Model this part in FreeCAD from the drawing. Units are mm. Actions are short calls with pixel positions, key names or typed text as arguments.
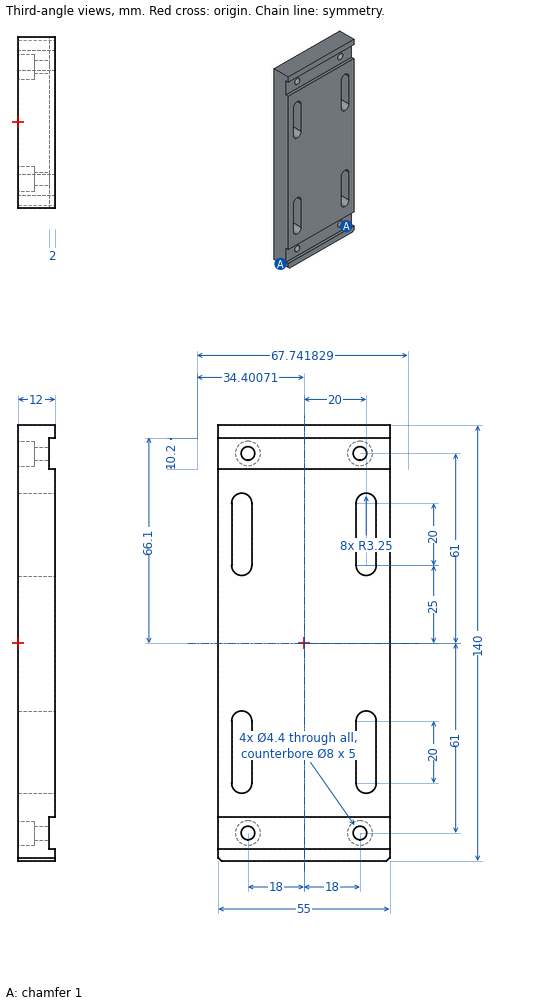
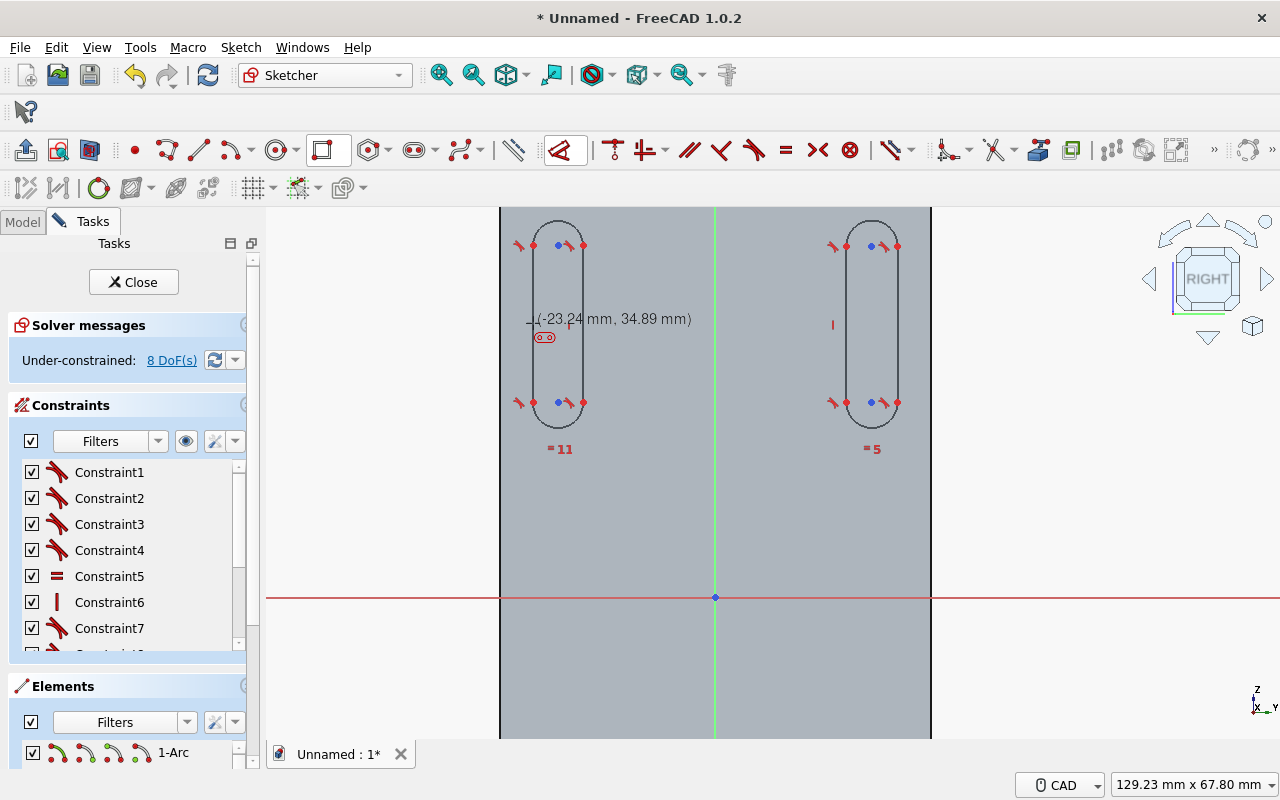
scroll(696, 371, down, 4)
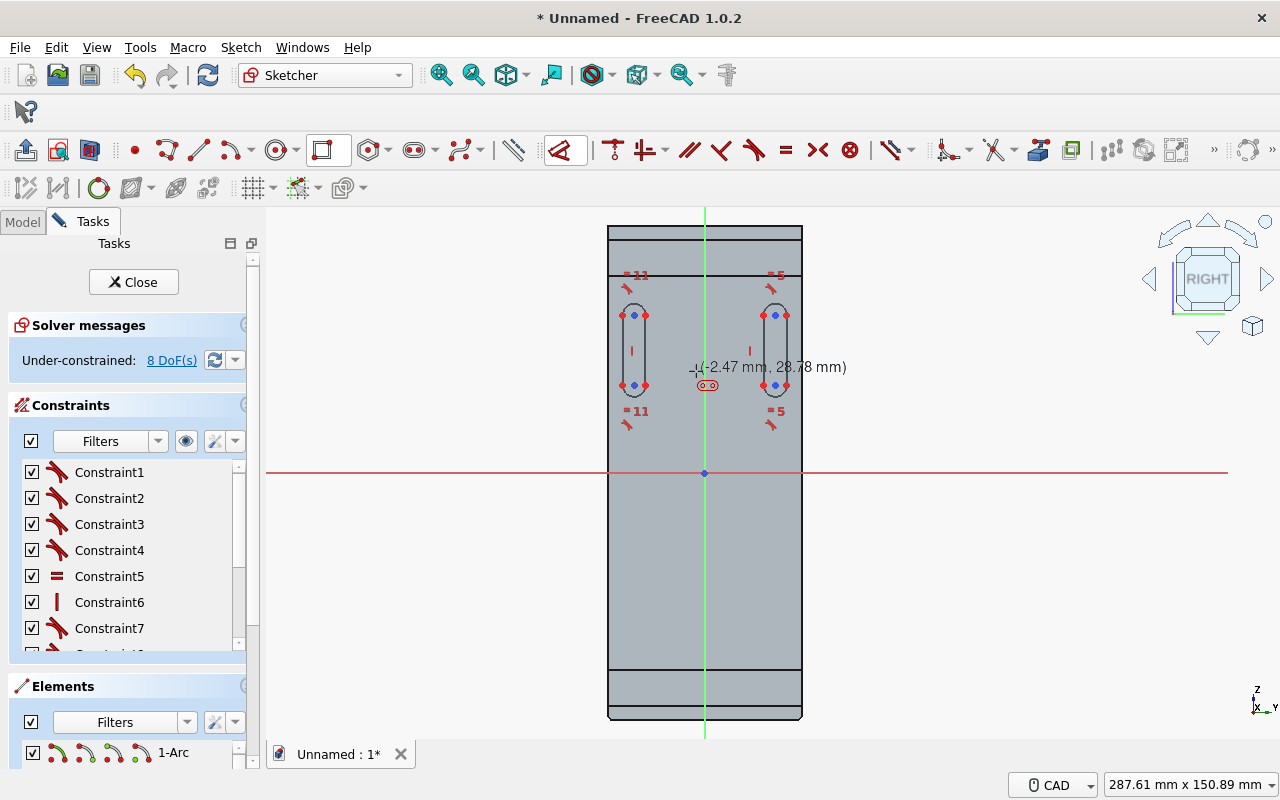
scroll(775, 632, up, 4)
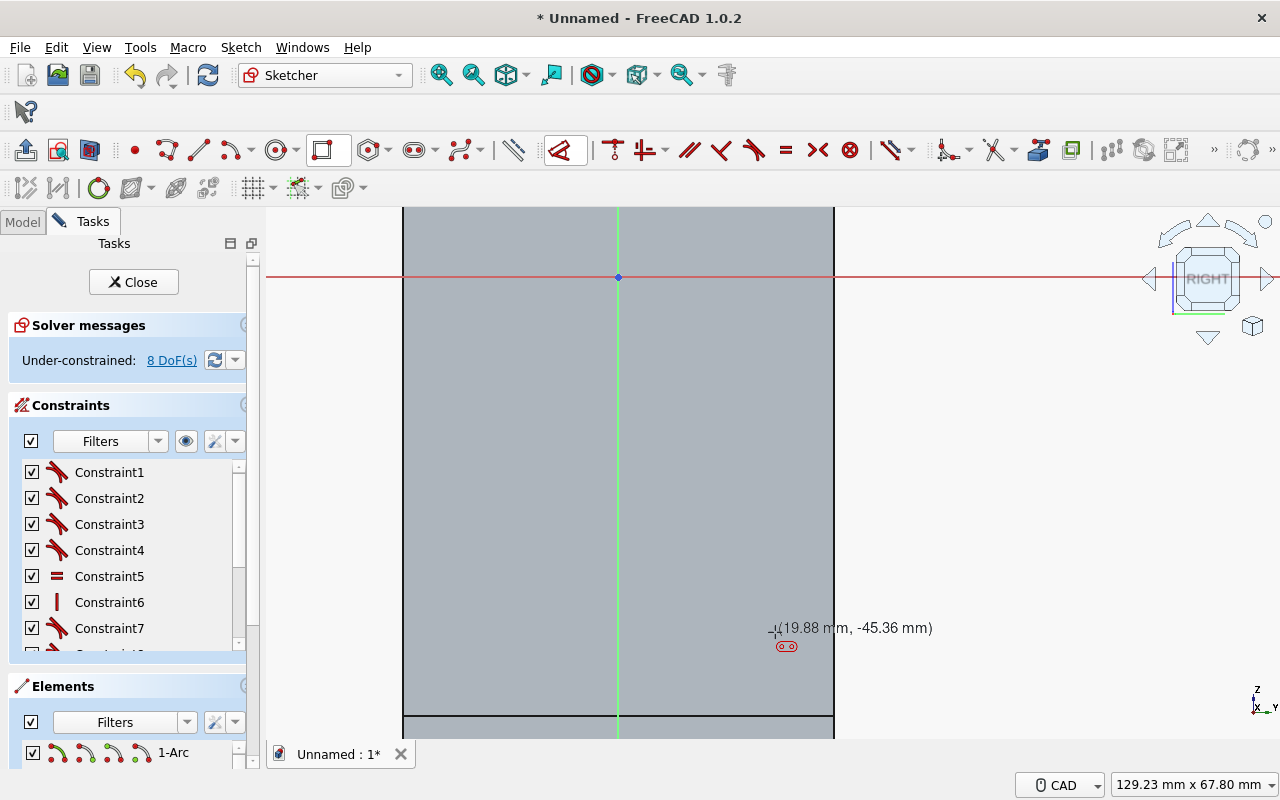
click(775, 630)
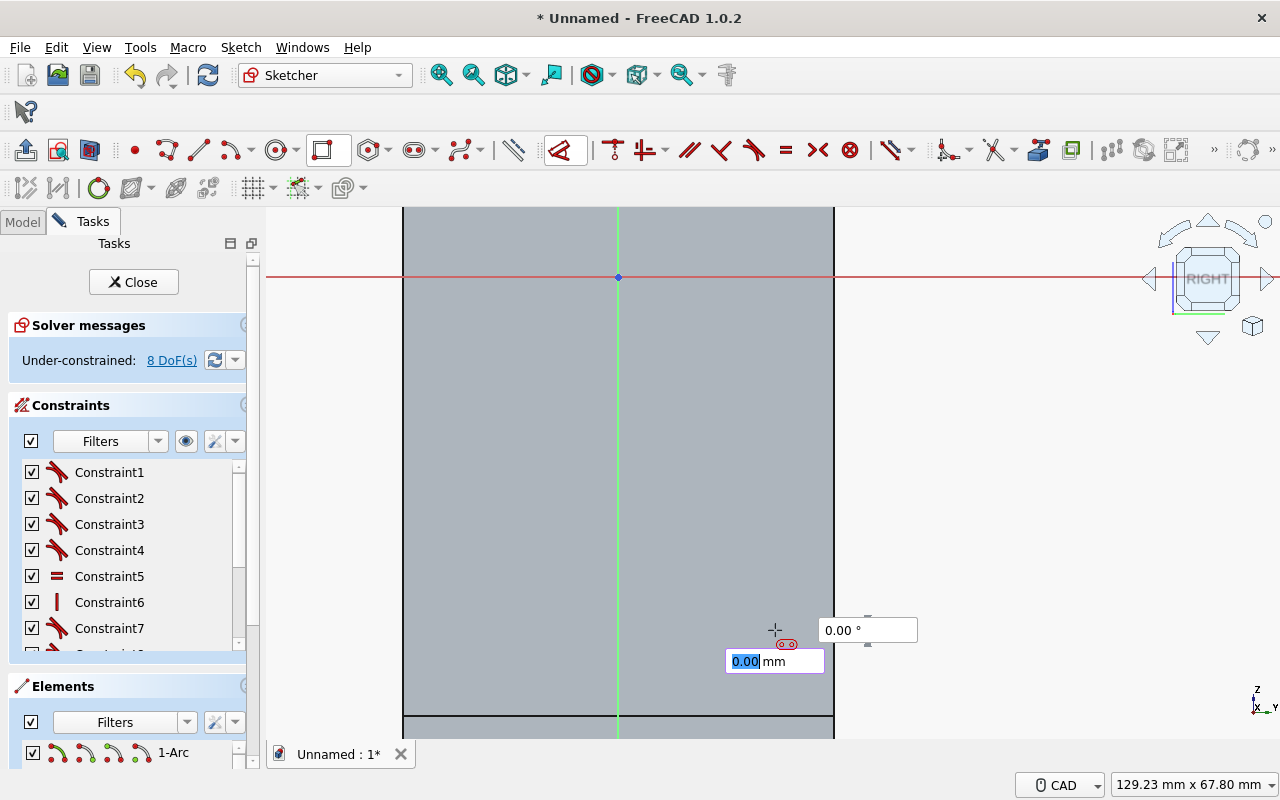
click(775, 473)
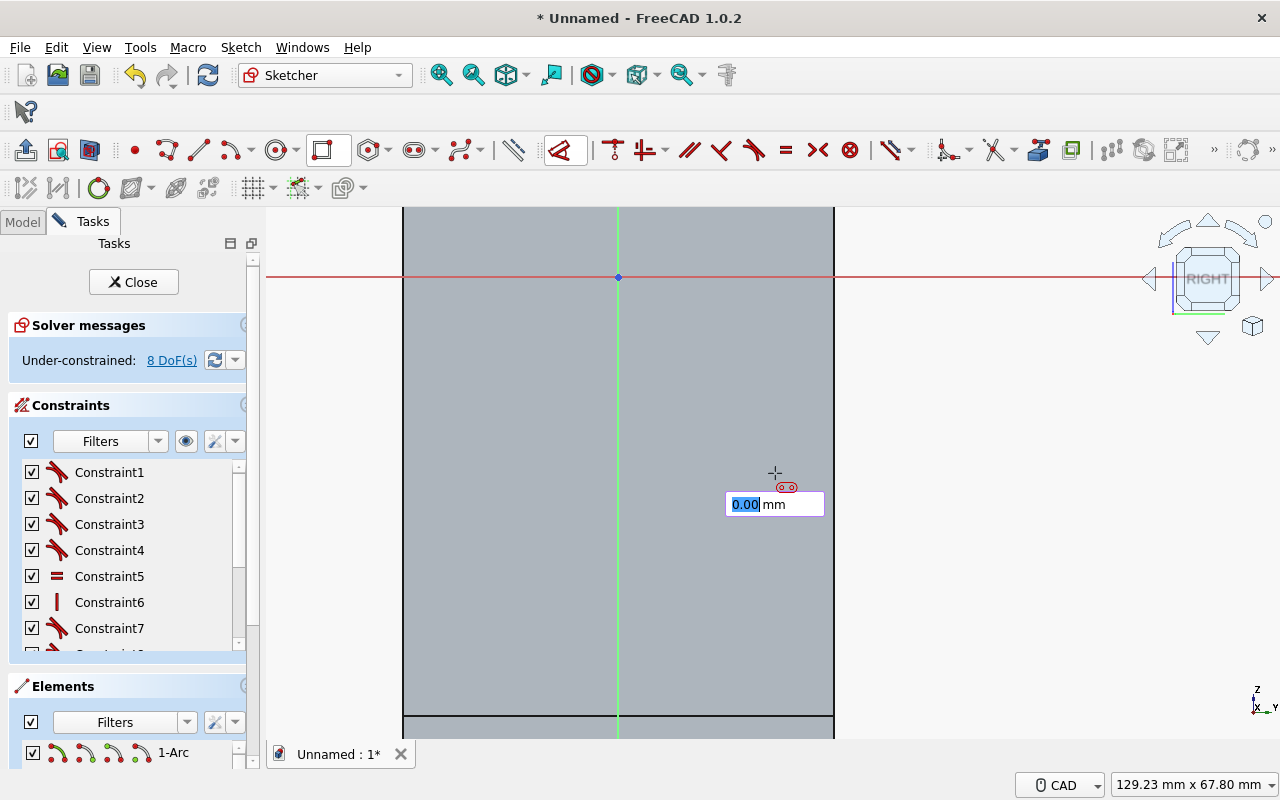
click(801, 552)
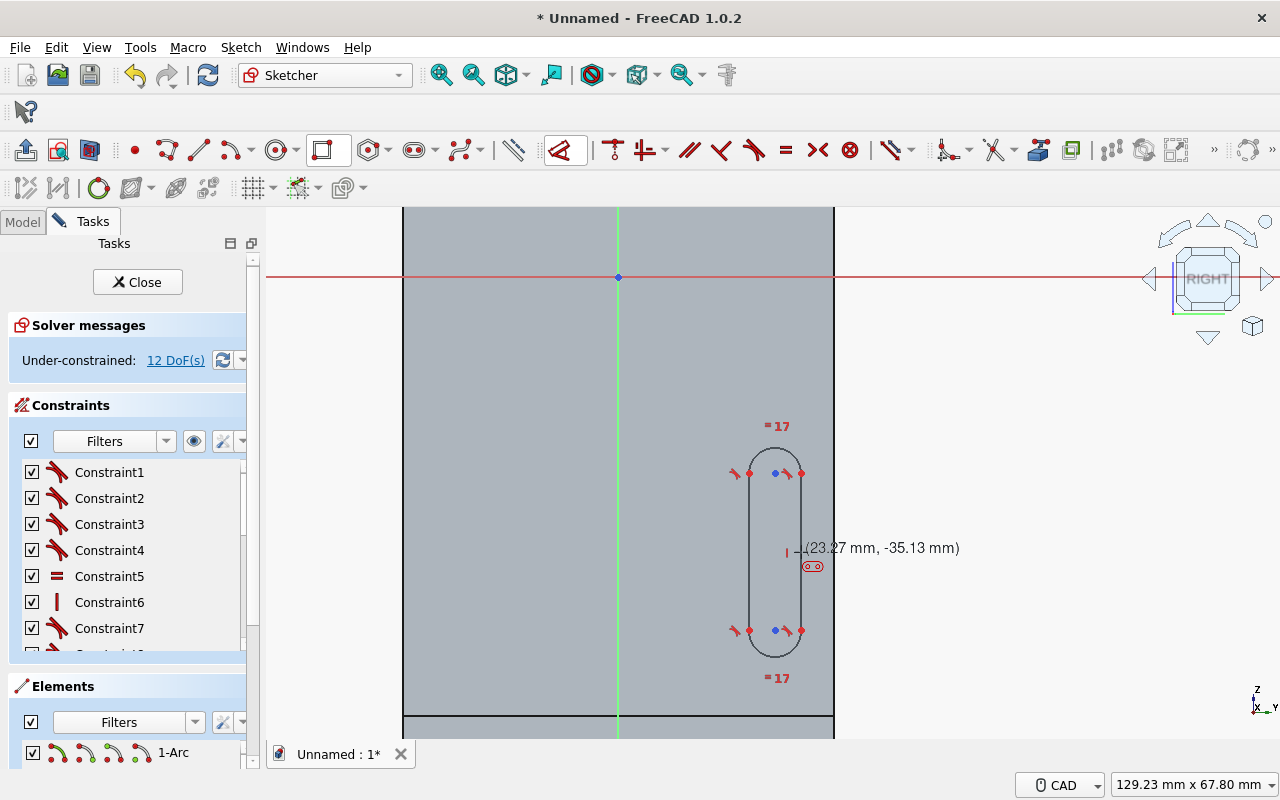
click(461, 630)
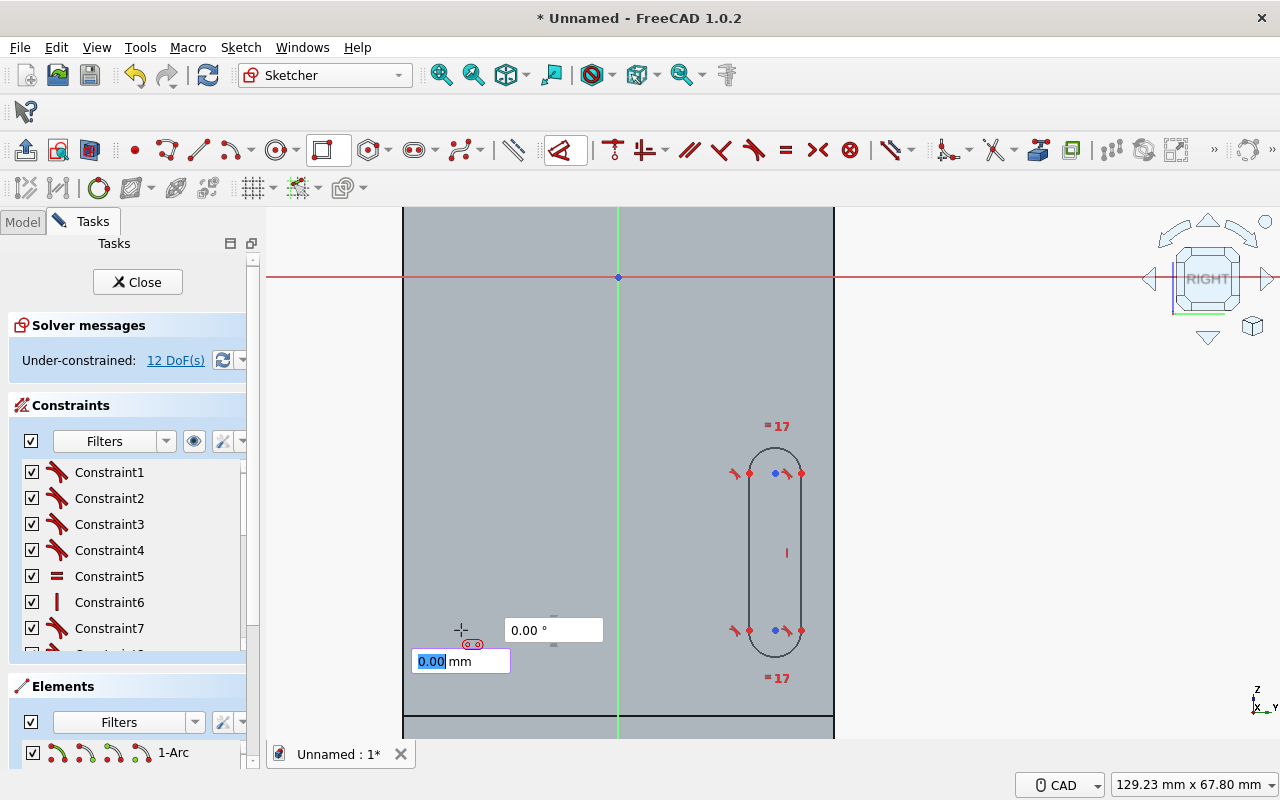
click(461, 473)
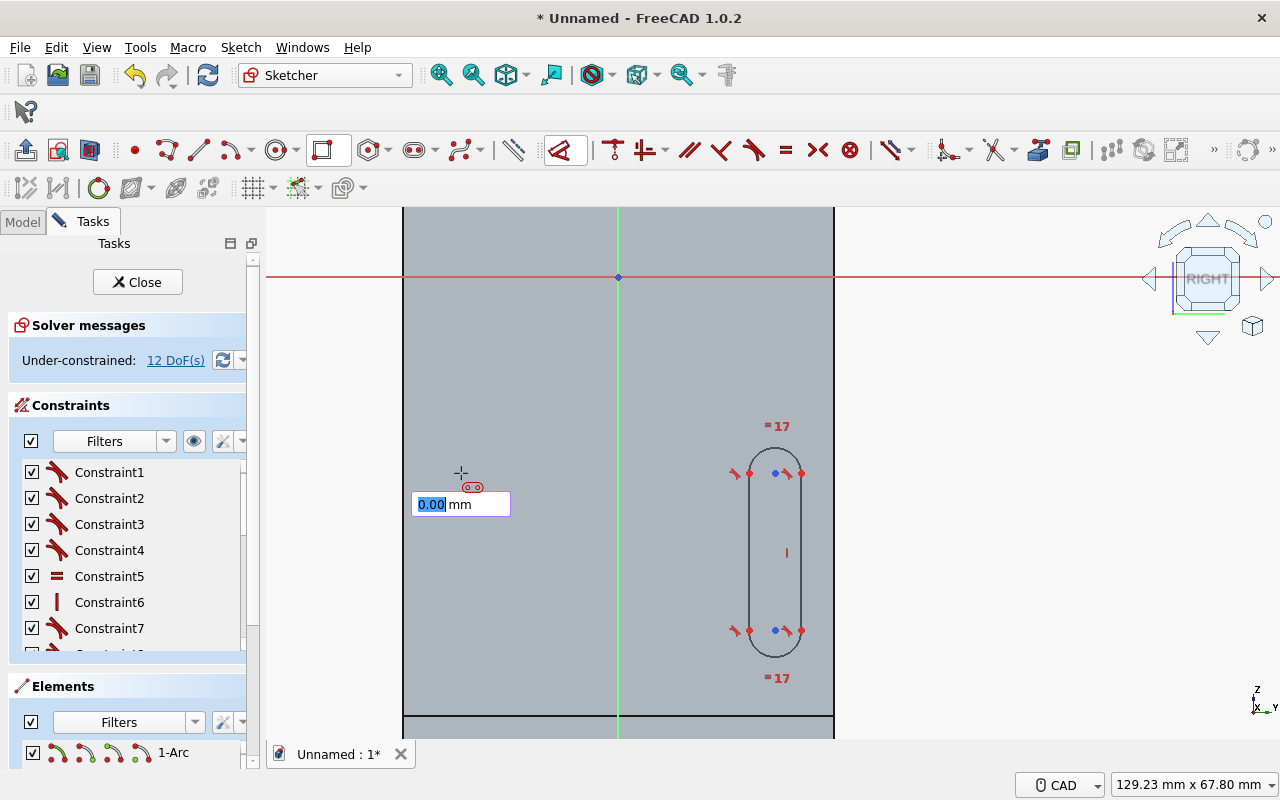
click(436, 552)
key(Escape)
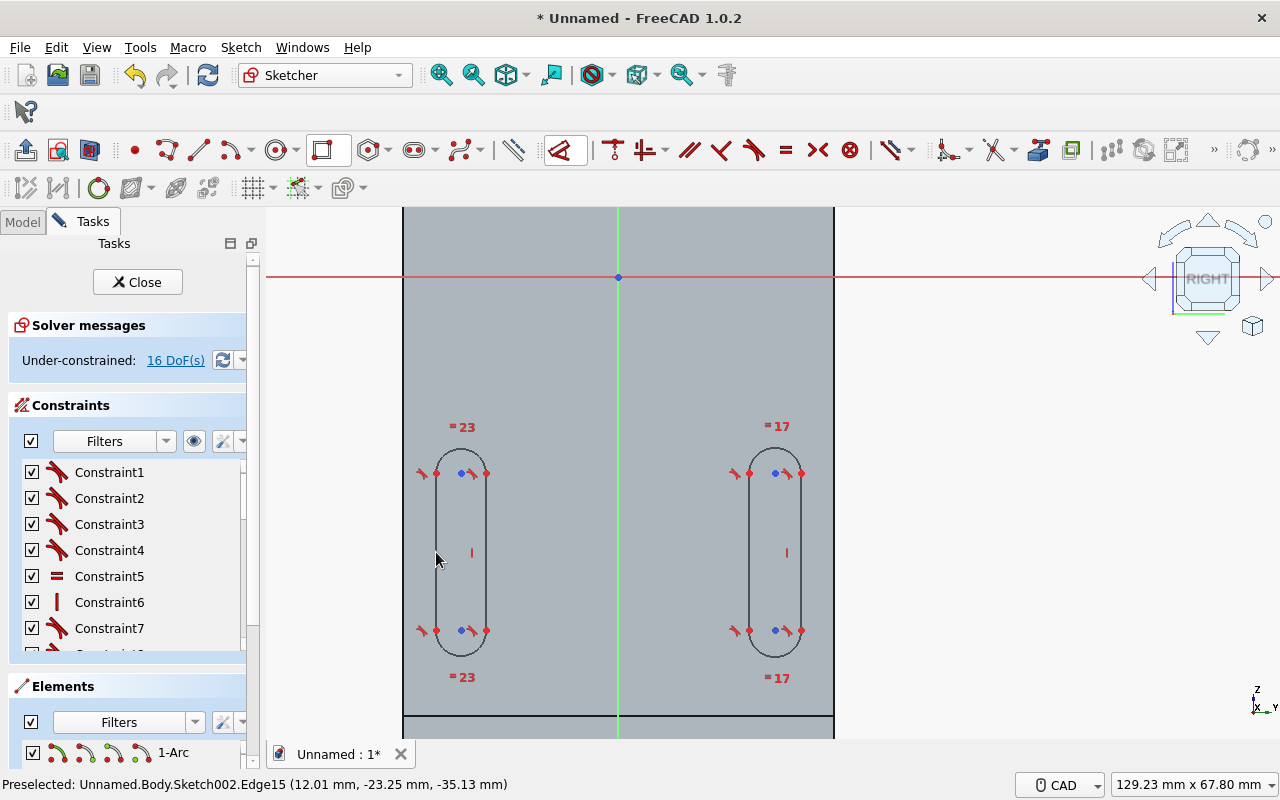
scroll(775, 633, down, 4)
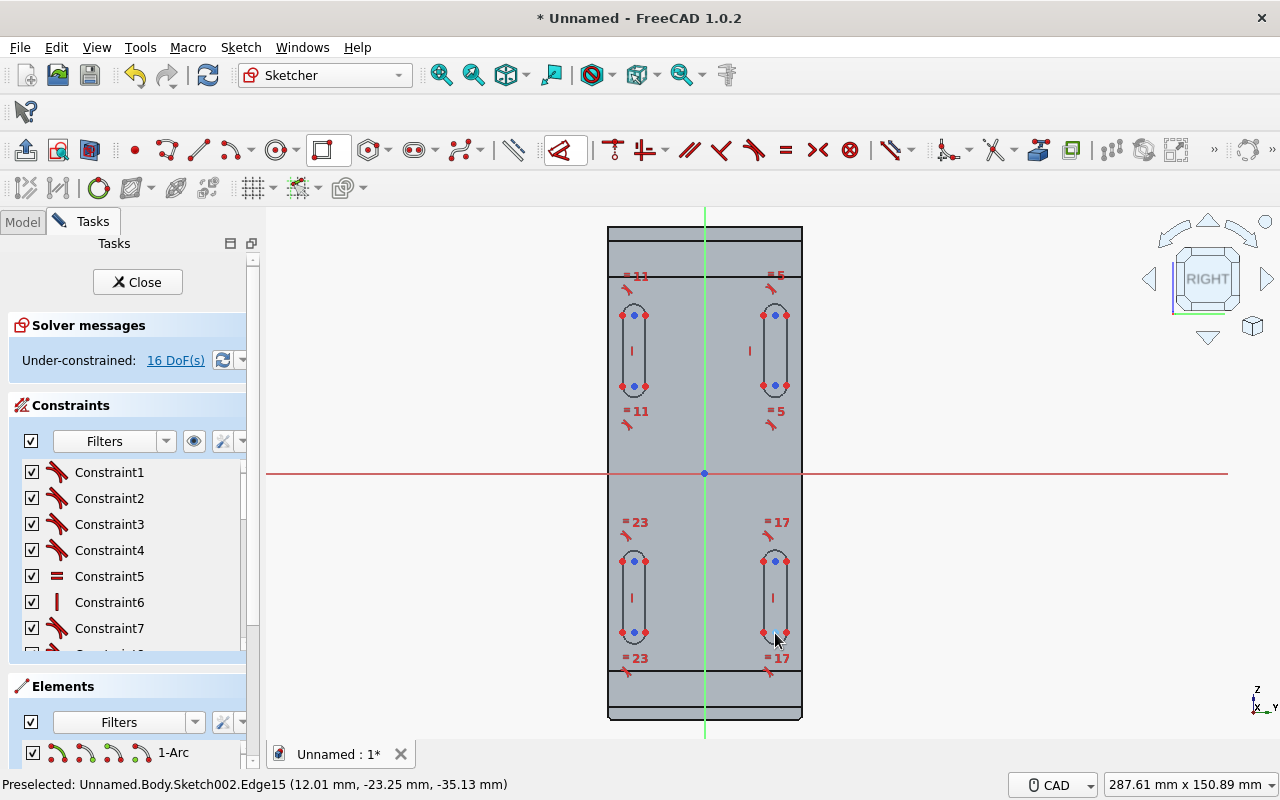
scroll(769, 395, up, 2)